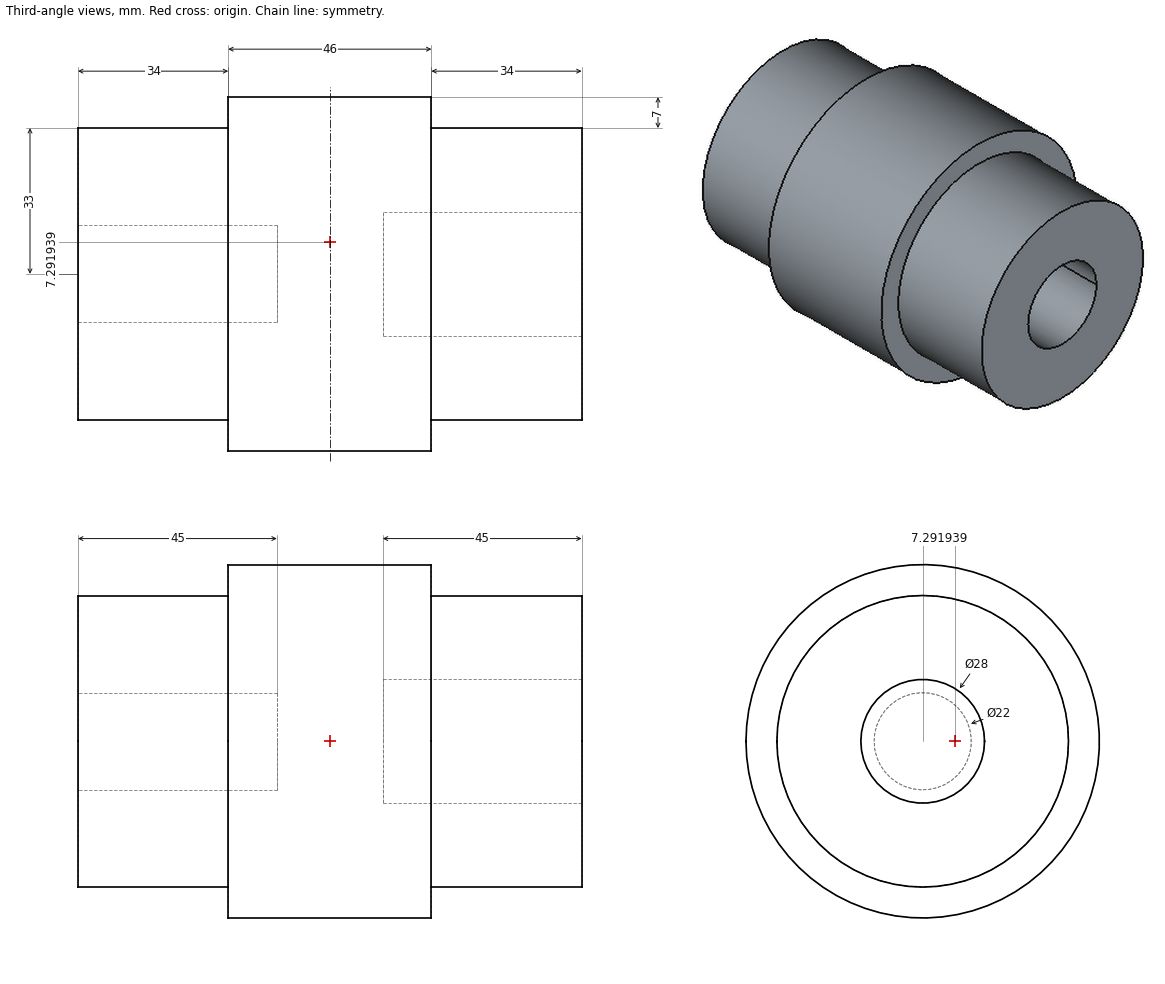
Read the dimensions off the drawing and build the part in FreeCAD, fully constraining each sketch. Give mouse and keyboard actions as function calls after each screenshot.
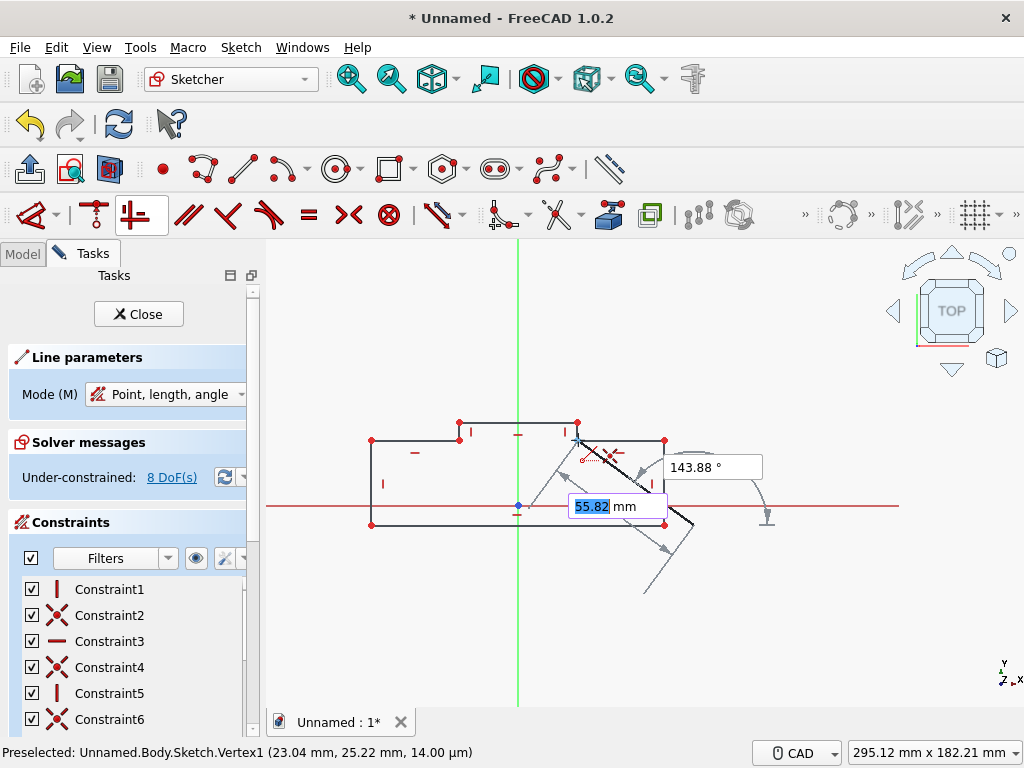
click(782, 525)
key(Escape)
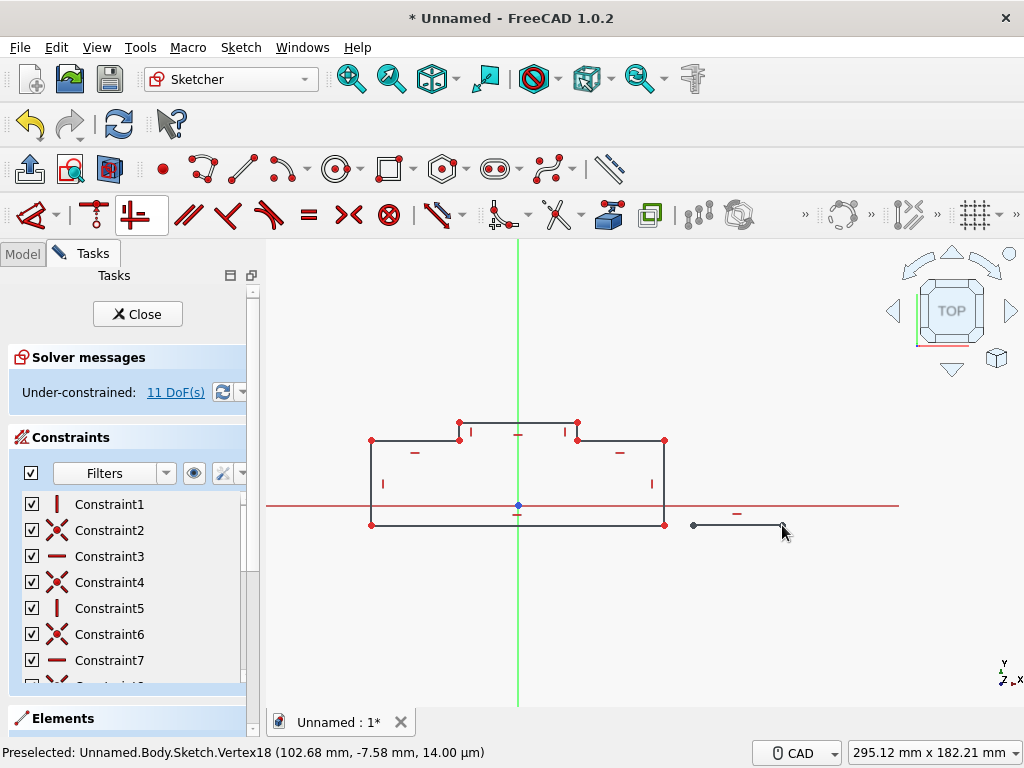
click(720, 525)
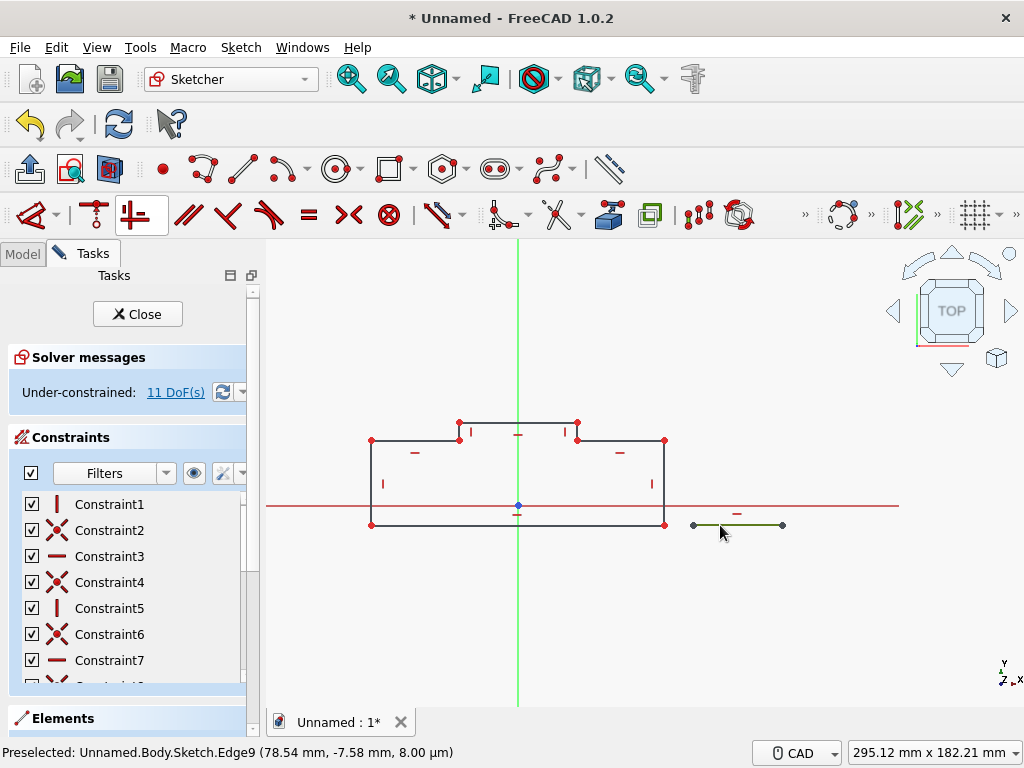
click(610, 170)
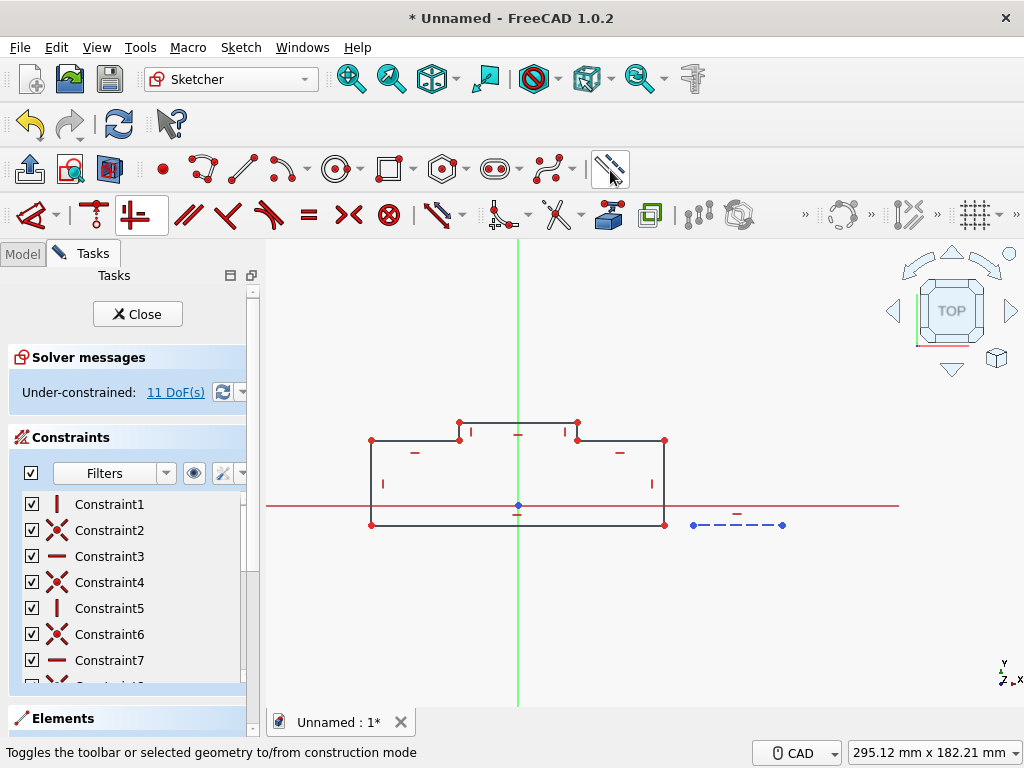
click(577, 441)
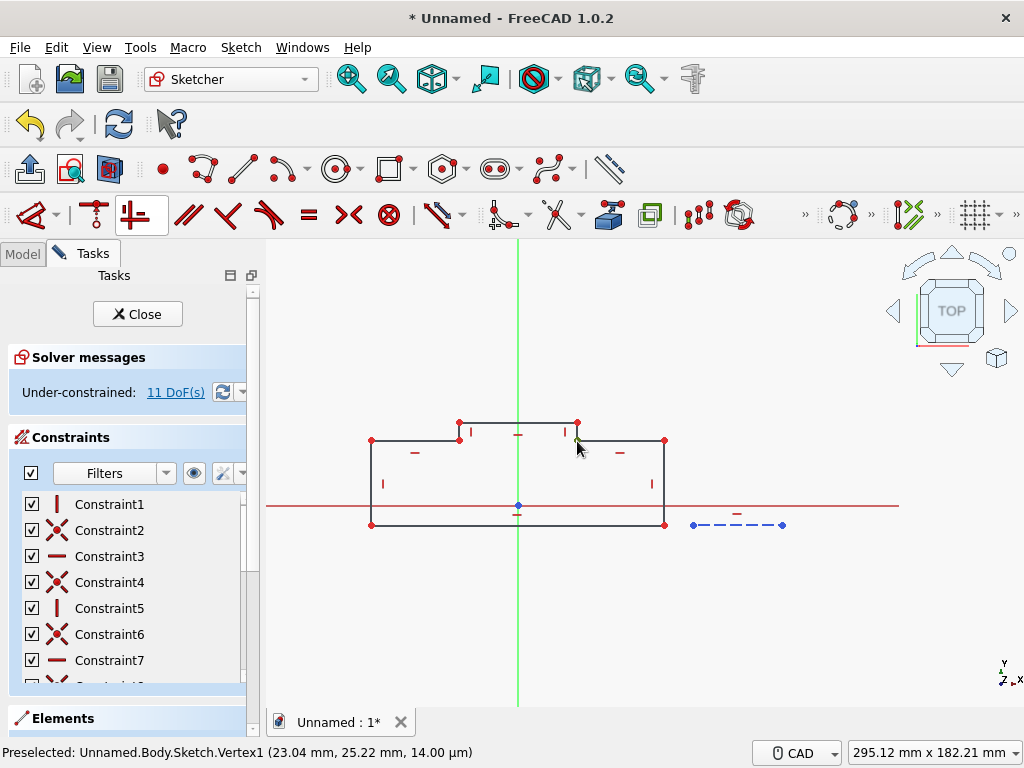
click(459, 441)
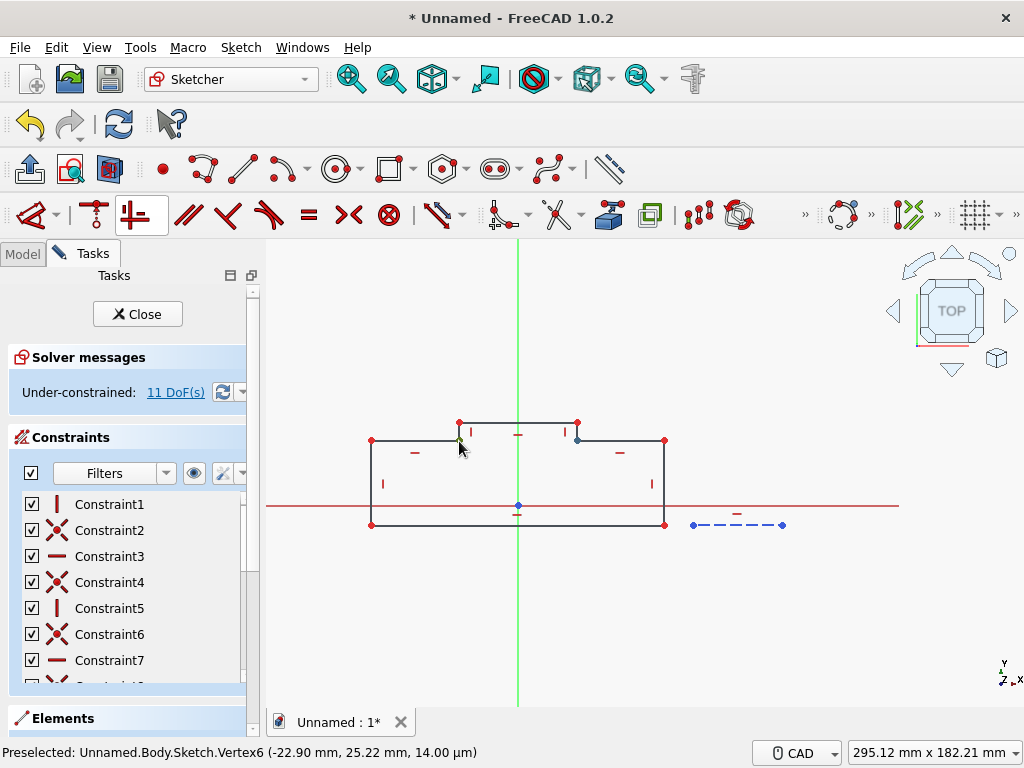
click(518, 650)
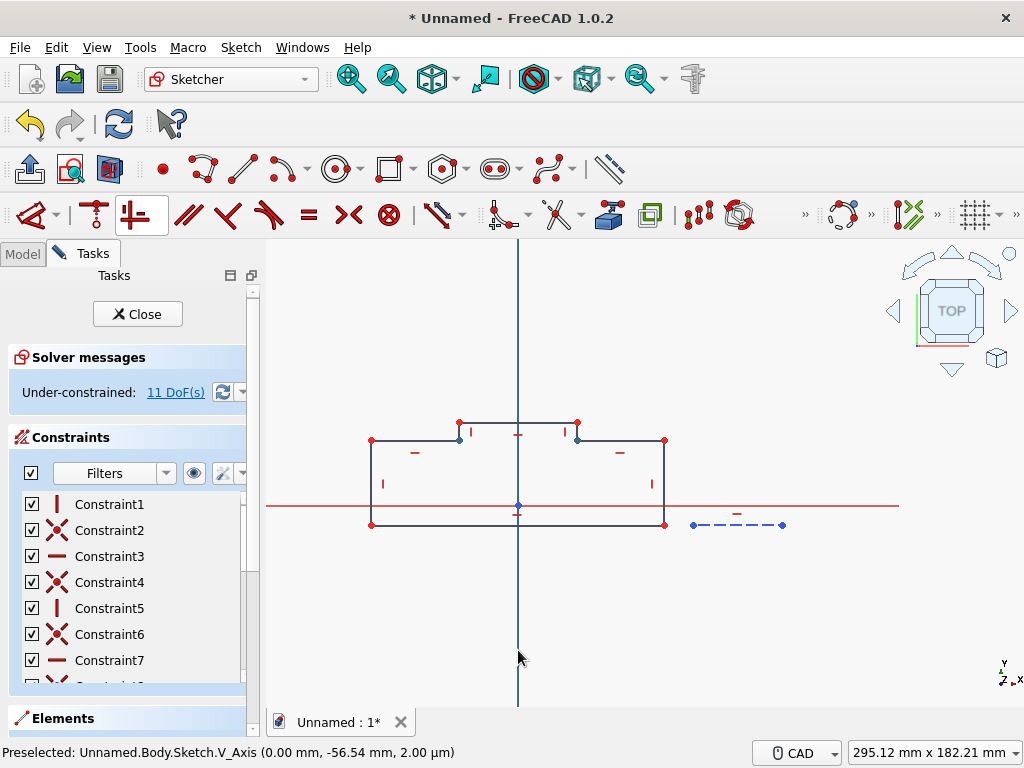
click(350, 216)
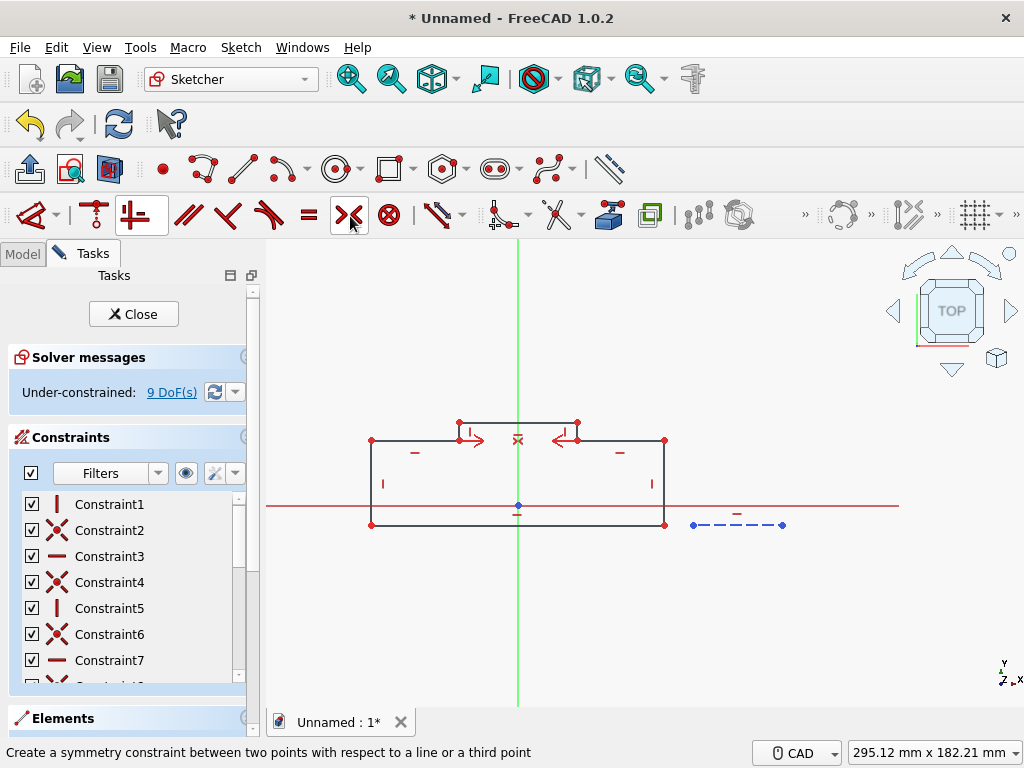
click(32, 216)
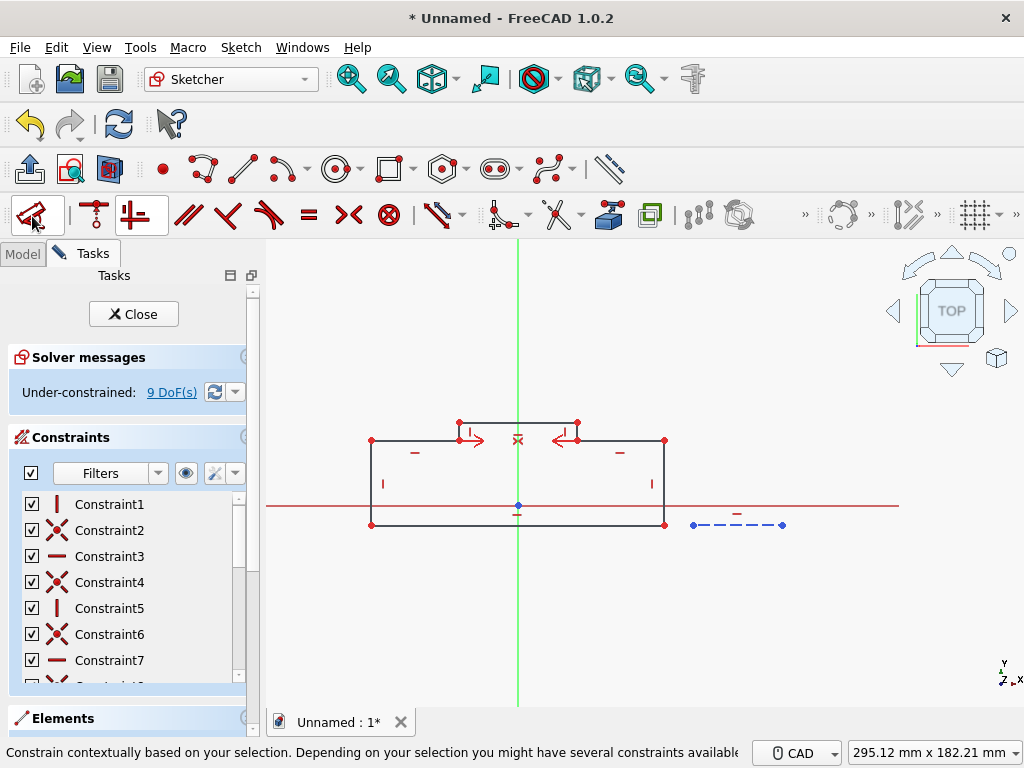
scroll(577, 432, up, 4)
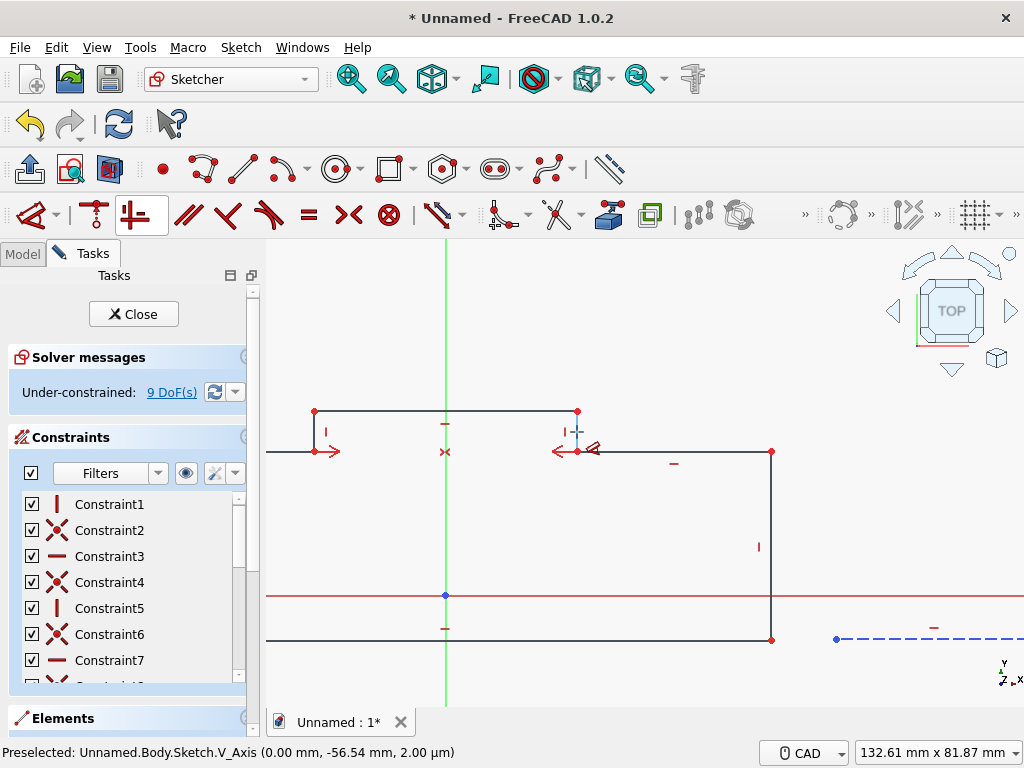
click(577, 431)
click(611, 431)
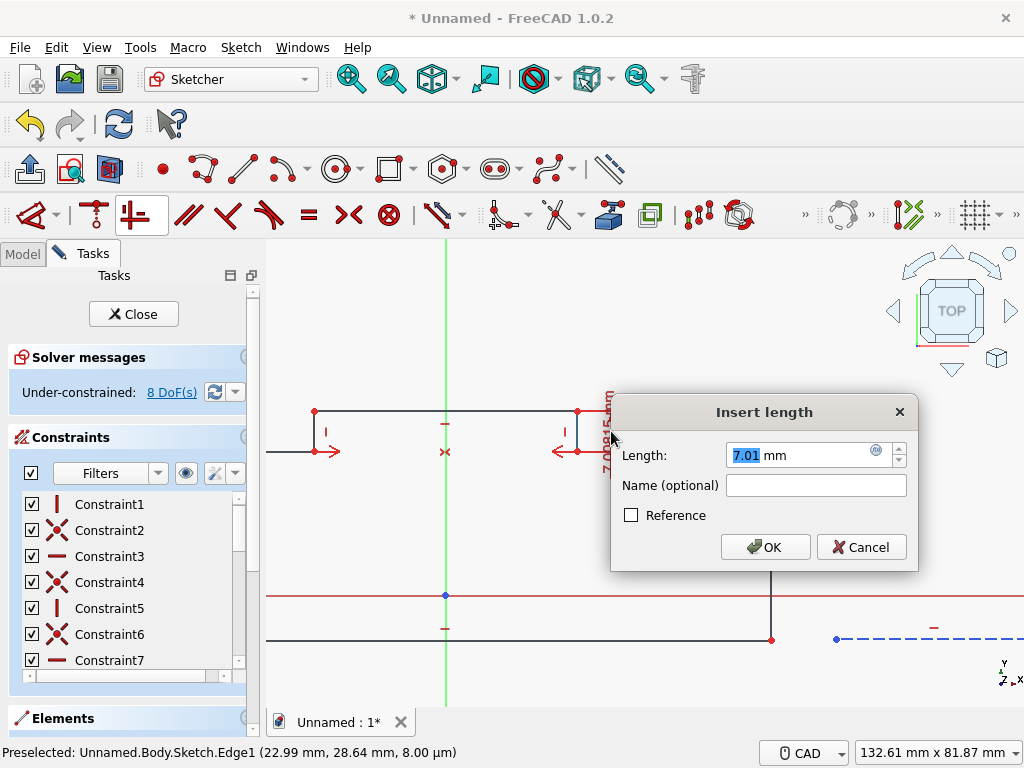
text(7)
key(Return)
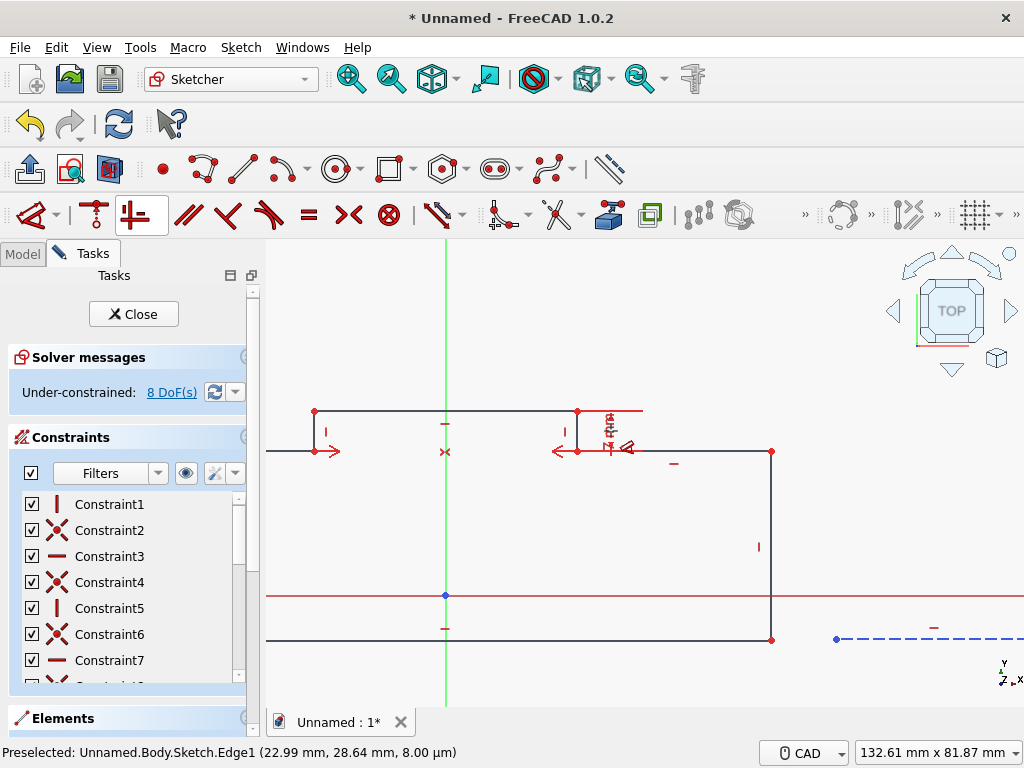
click(498, 411)
click(385, 377)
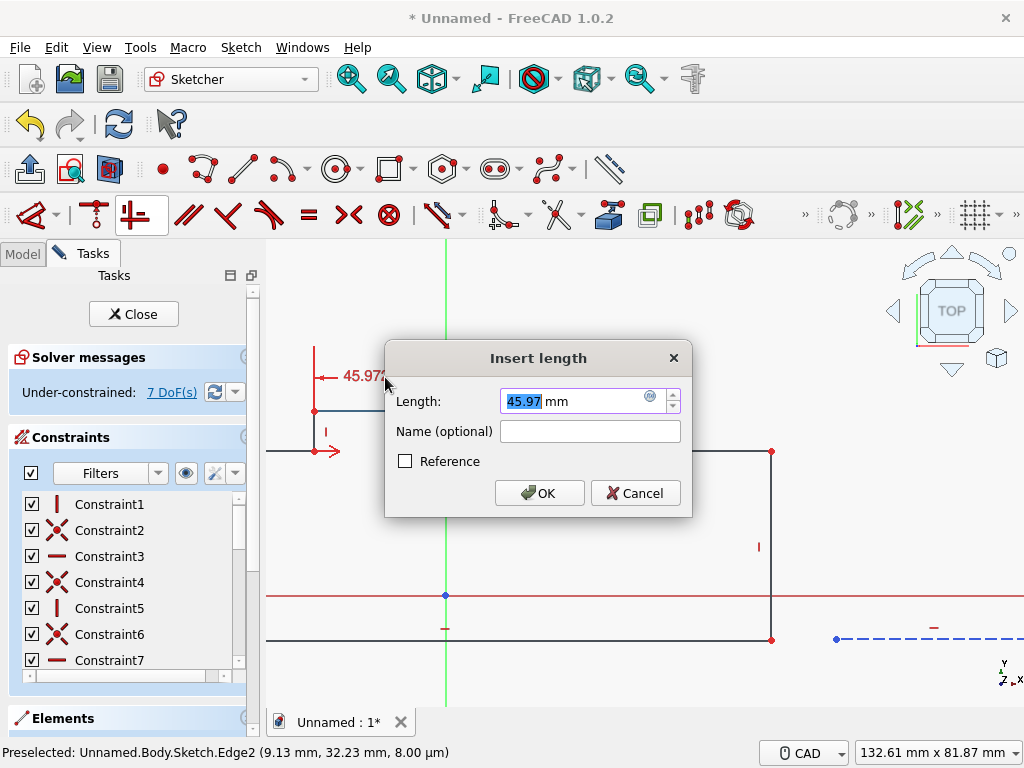
text(46)
key(Return)